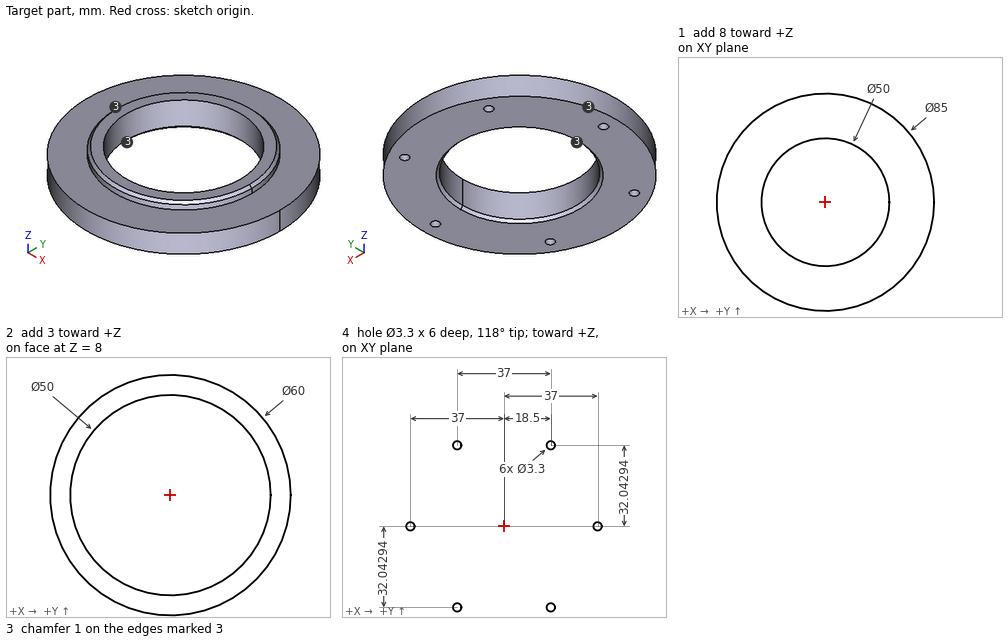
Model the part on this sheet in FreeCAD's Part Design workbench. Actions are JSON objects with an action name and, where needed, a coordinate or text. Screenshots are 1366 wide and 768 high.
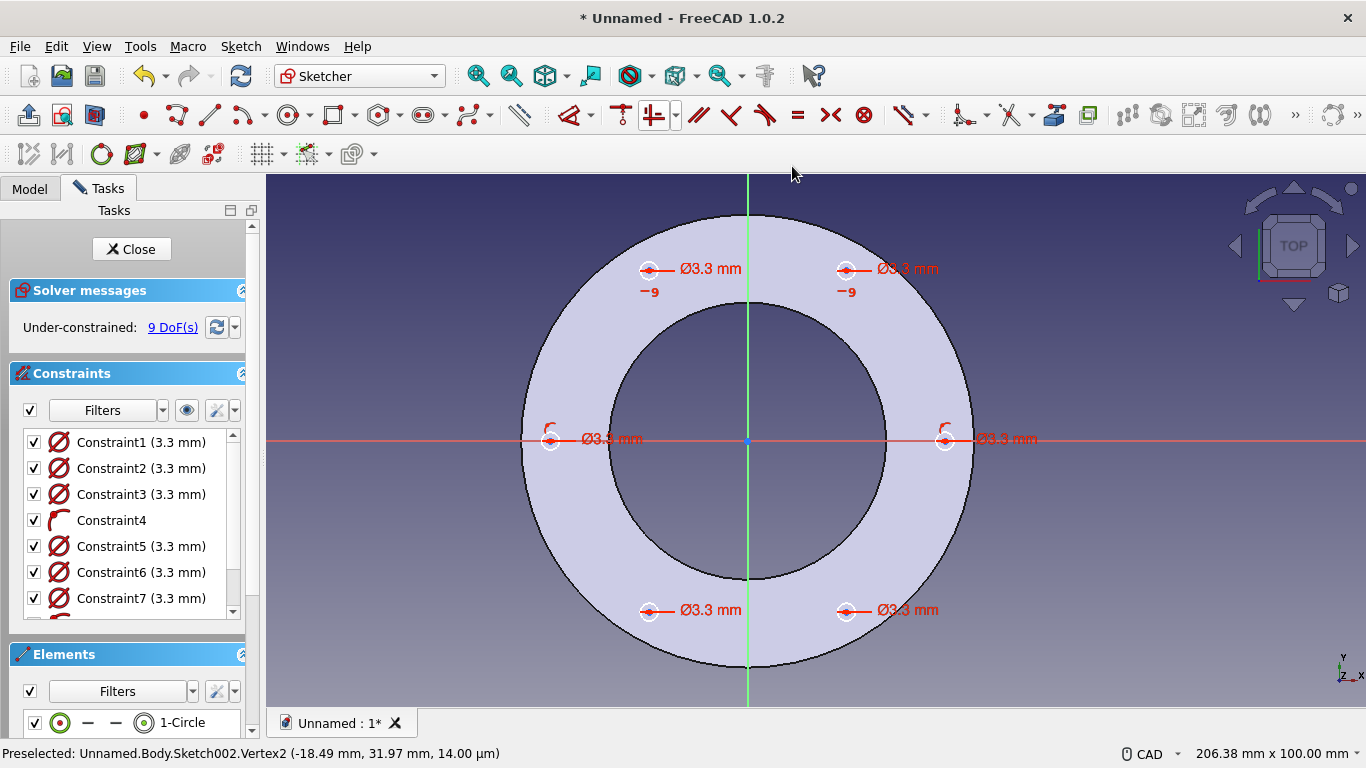
{"action": "left_click", "coordinate": [649, 271]}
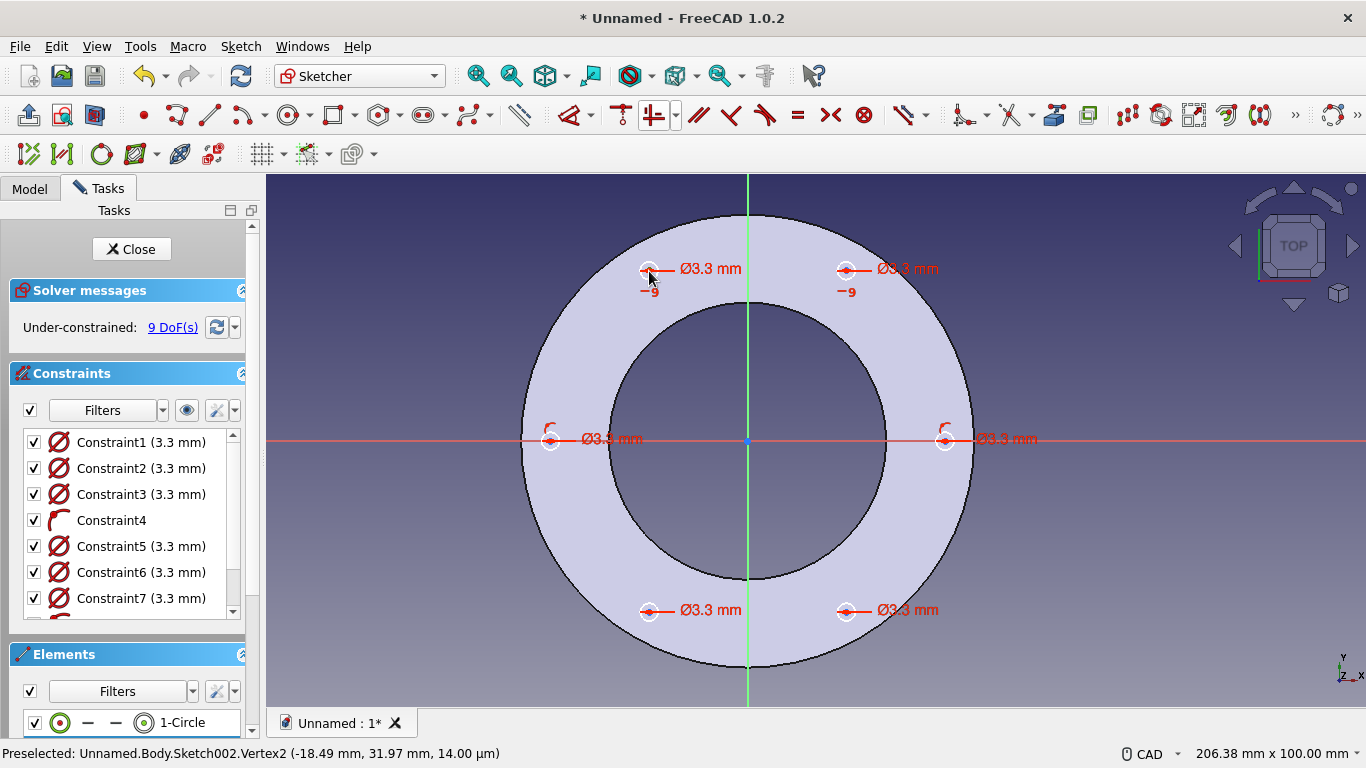
{"action": "left_click", "coordinate": [649, 612]}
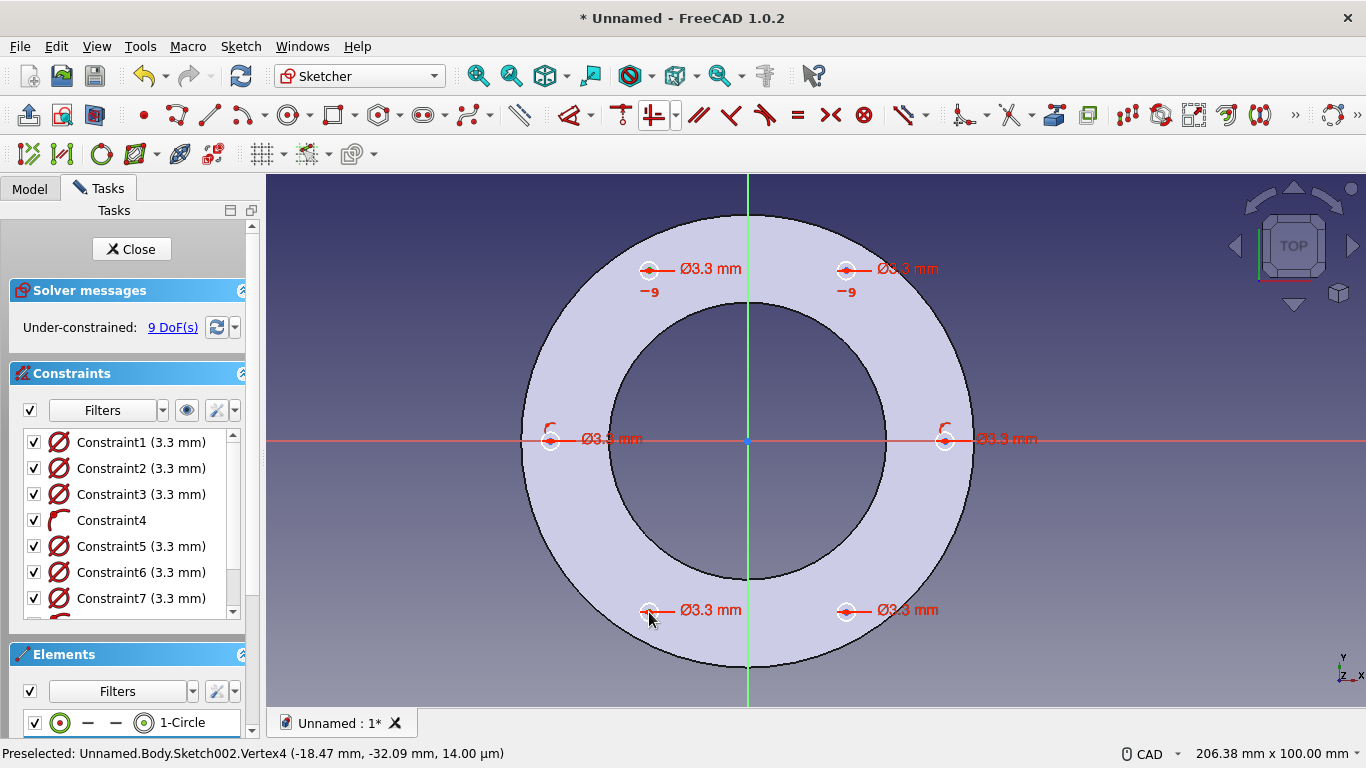
{"action": "left_click", "coordinate": [676, 116]}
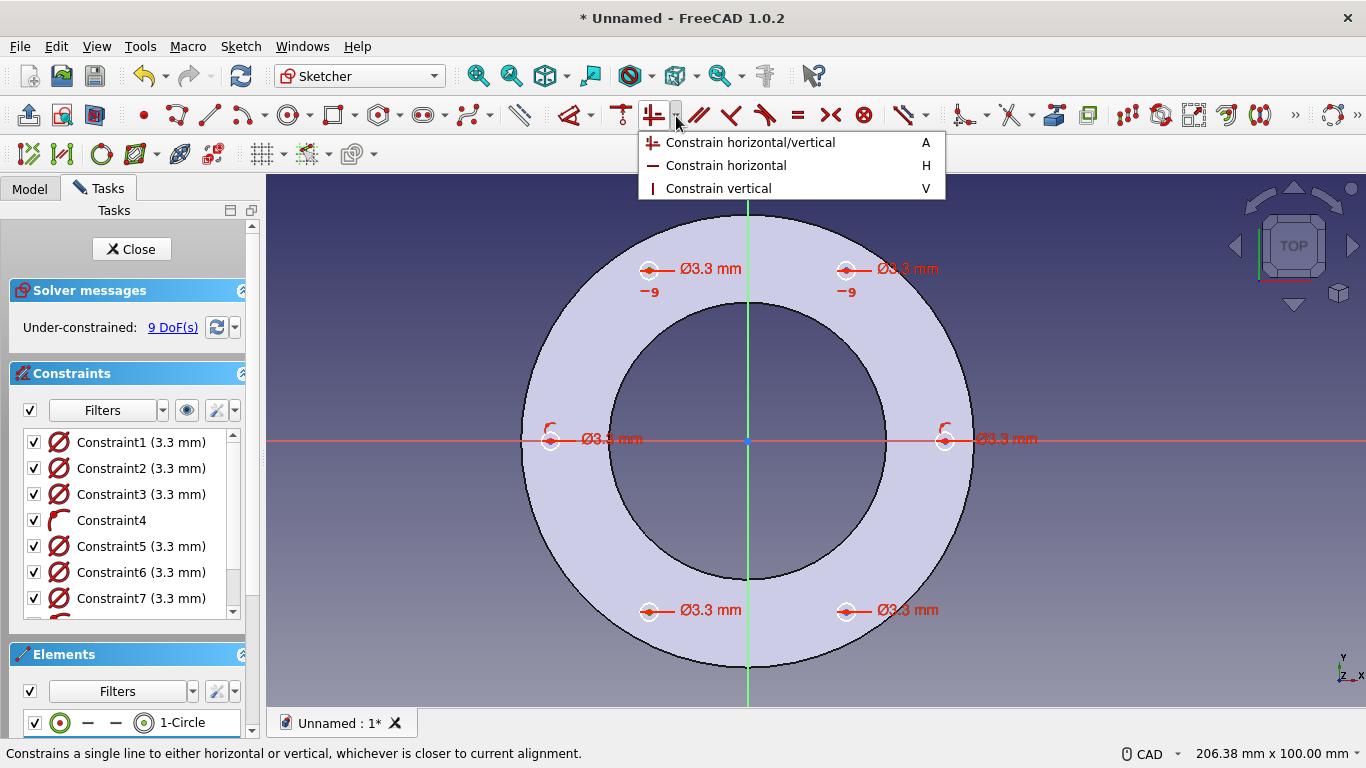
{"action": "left_click", "coordinate": [792, 188]}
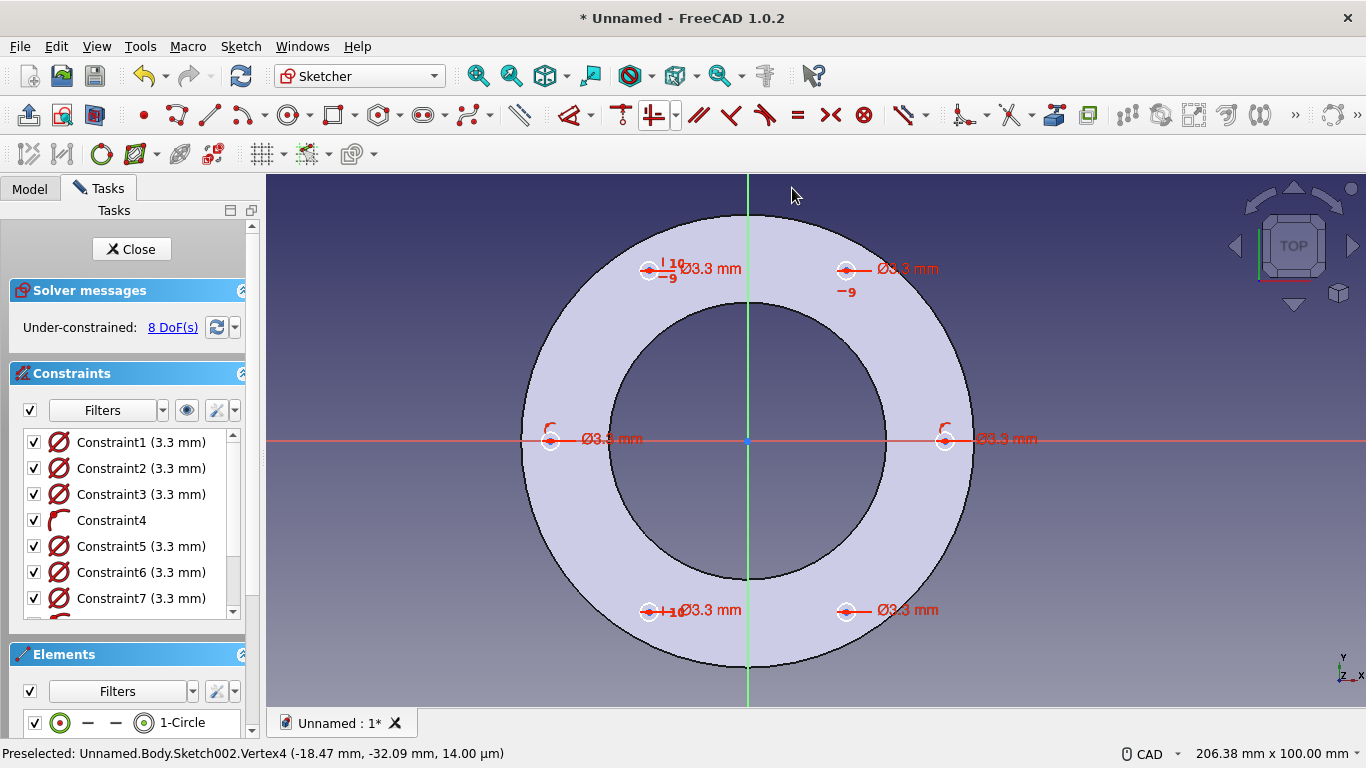
{"action": "left_click", "coordinate": [846, 271]}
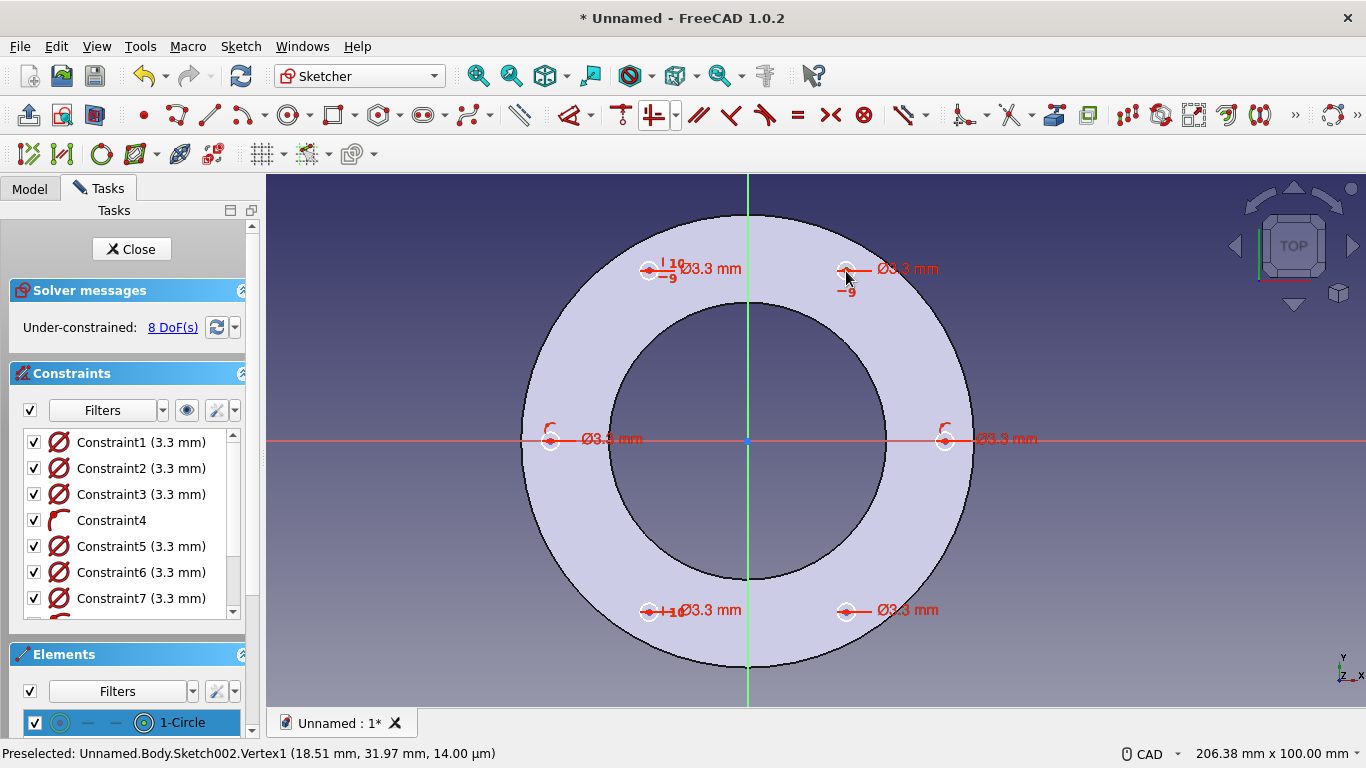
{"action": "left_click", "coordinate": [846, 612]}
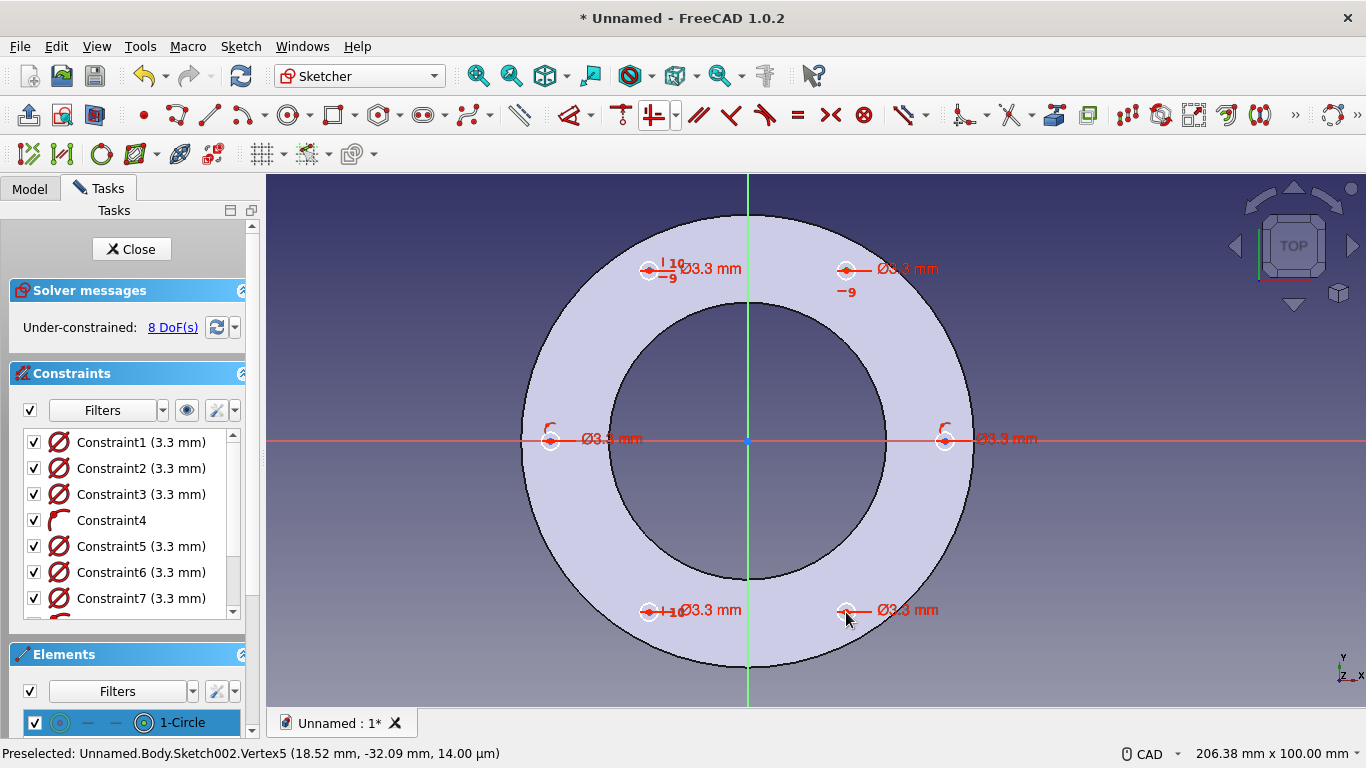
{"action": "left_click", "coordinate": [676, 116]}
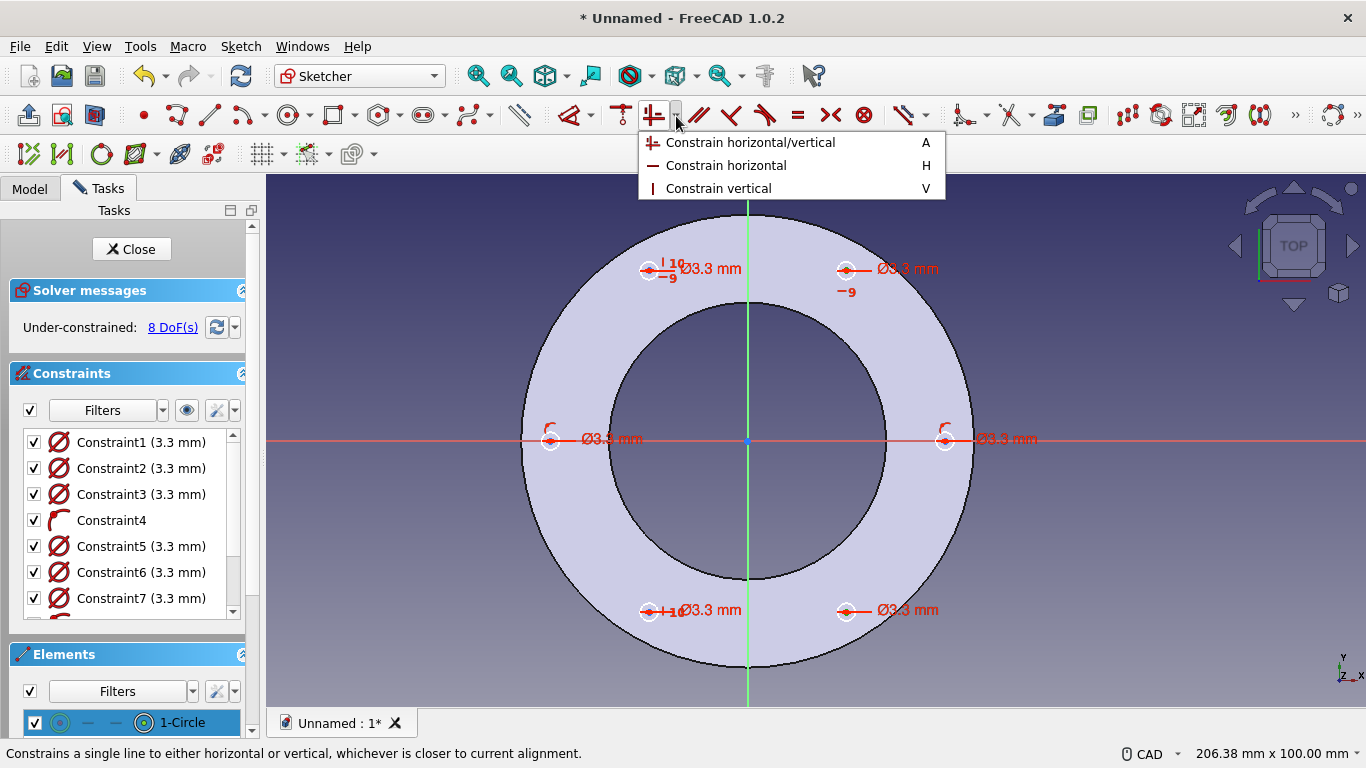
{"action": "left_click", "coordinate": [792, 188]}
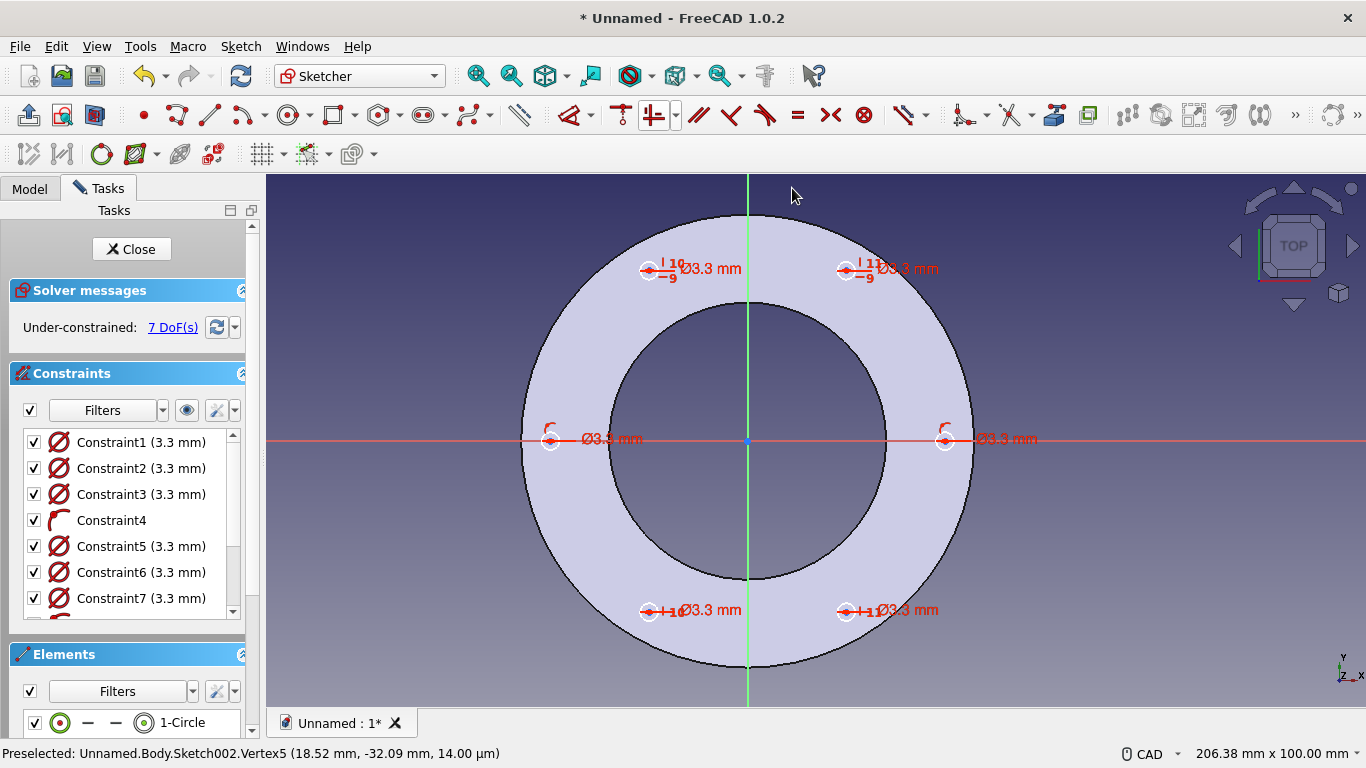
{"action": "left_click", "coordinate": [649, 612]}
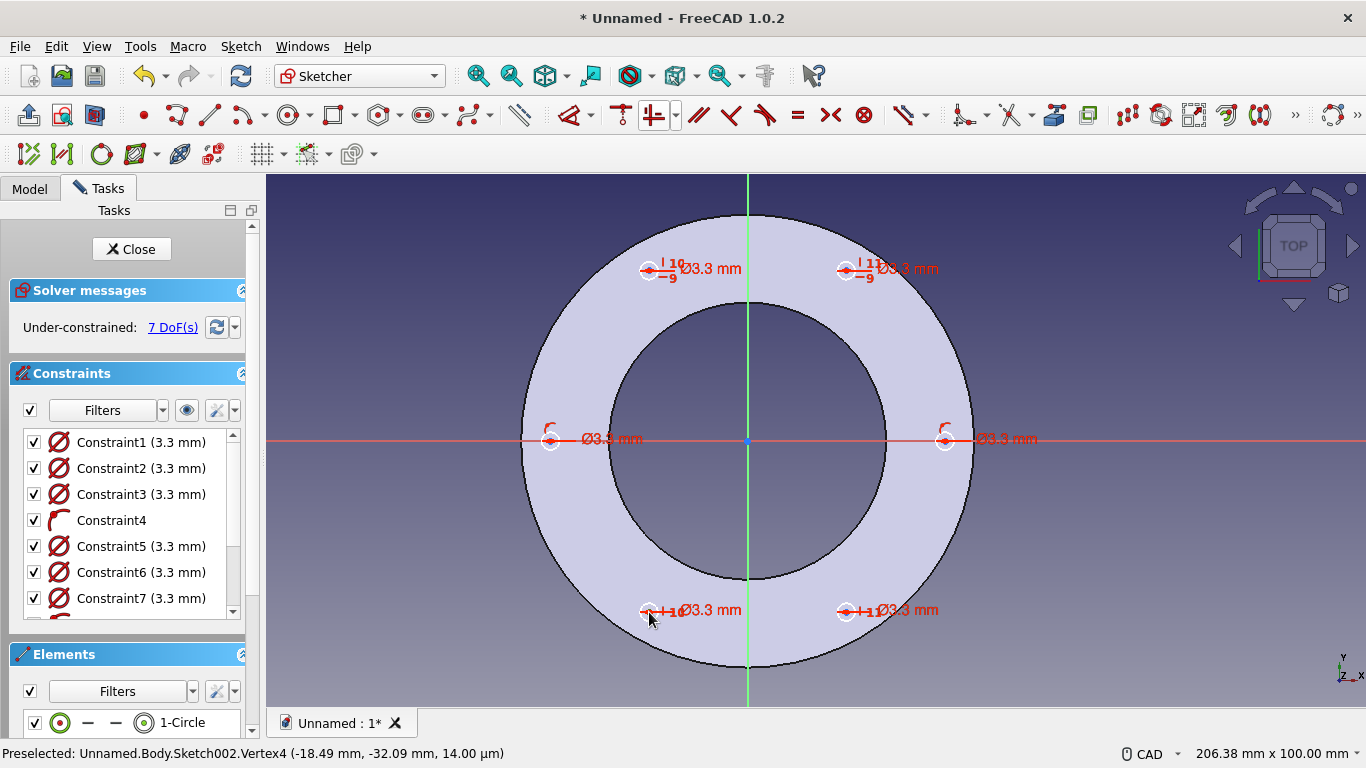
{"action": "left_click", "coordinate": [846, 612]}